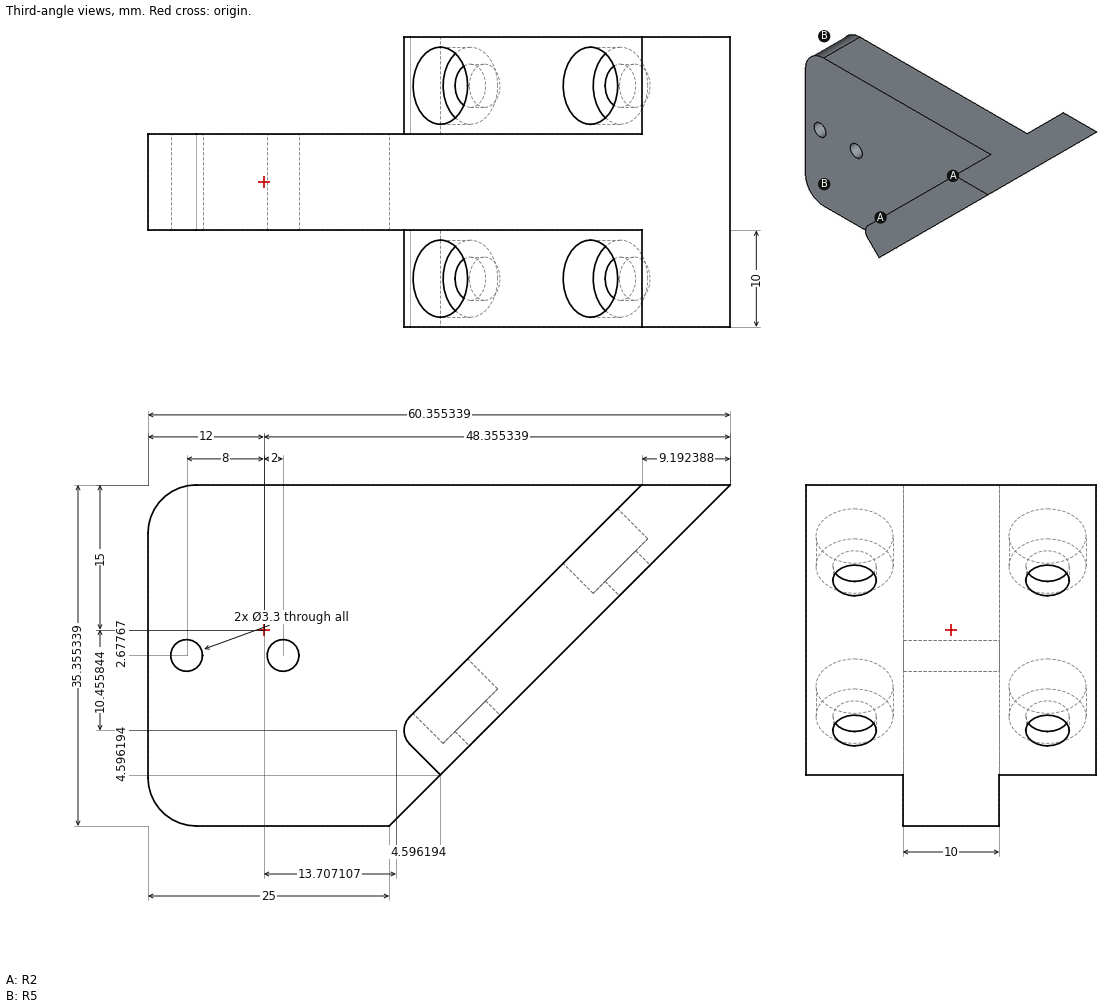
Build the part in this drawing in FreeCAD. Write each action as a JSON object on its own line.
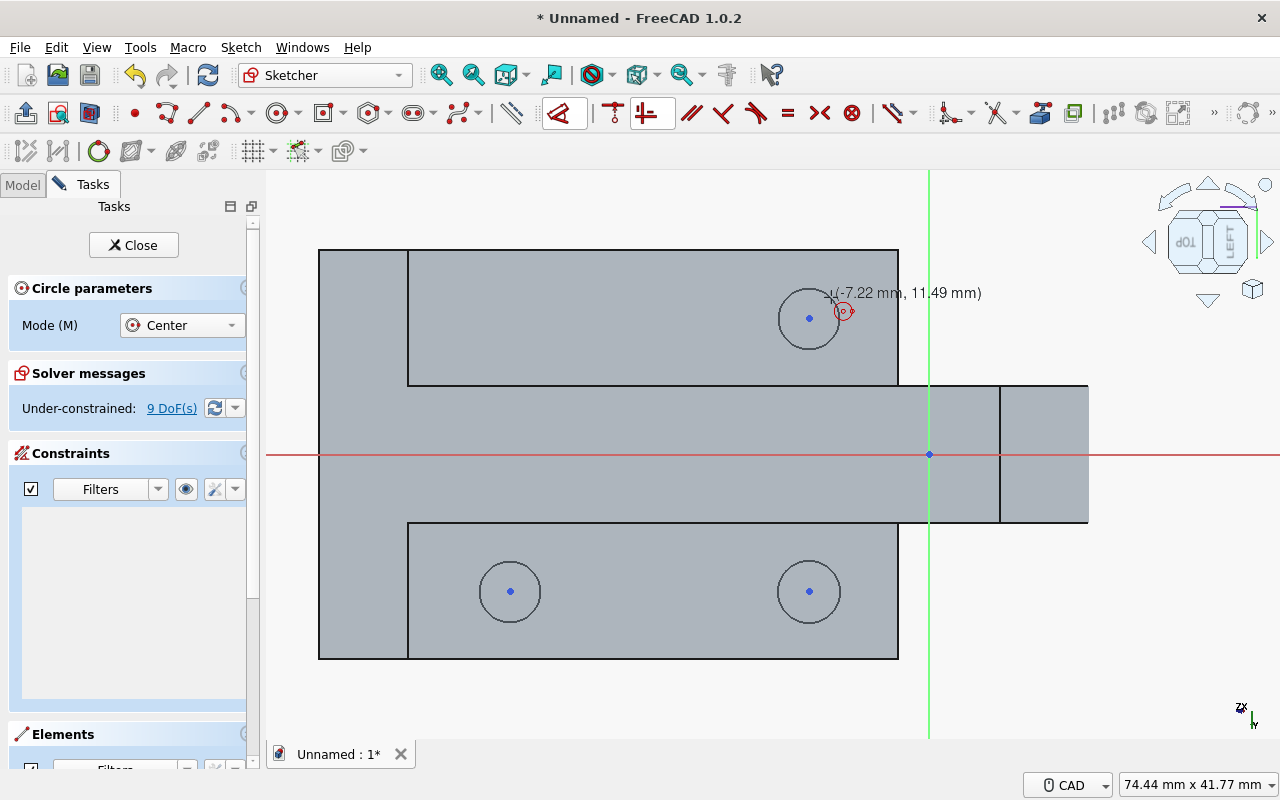
{"action": "left_click", "coordinate": [510, 318]}
{"action": "left_click", "coordinate": [531, 297]}
{"action": "key", "text": "Escape"}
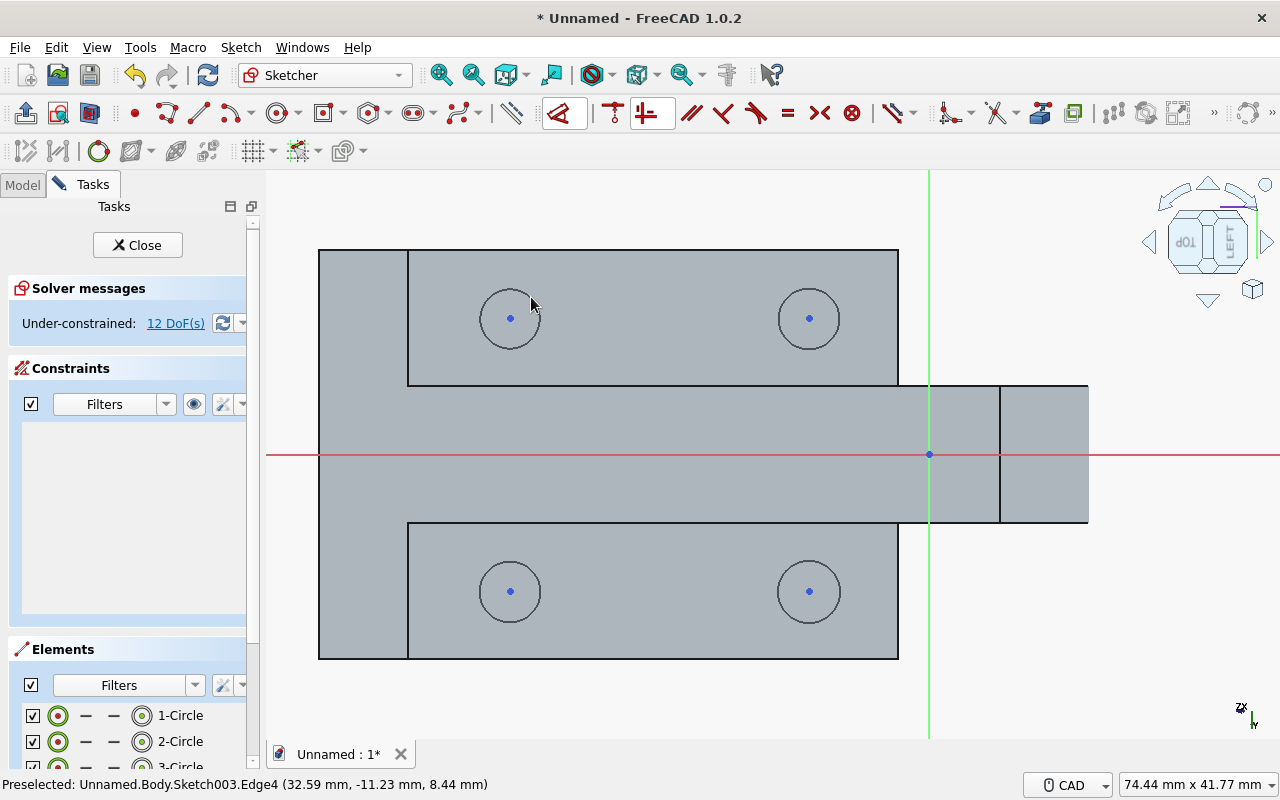
{"action": "left_click", "coordinate": [831, 570]}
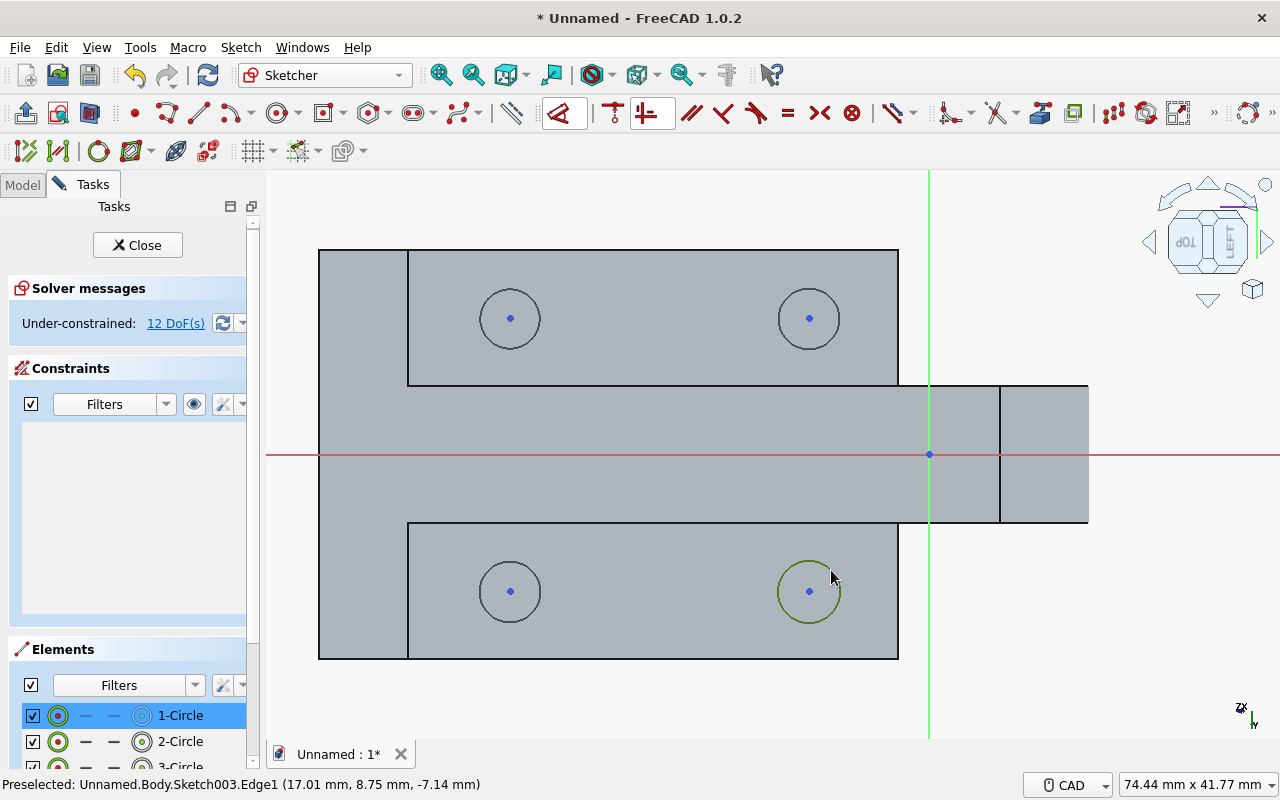
{"action": "left_click", "coordinate": [531, 570]}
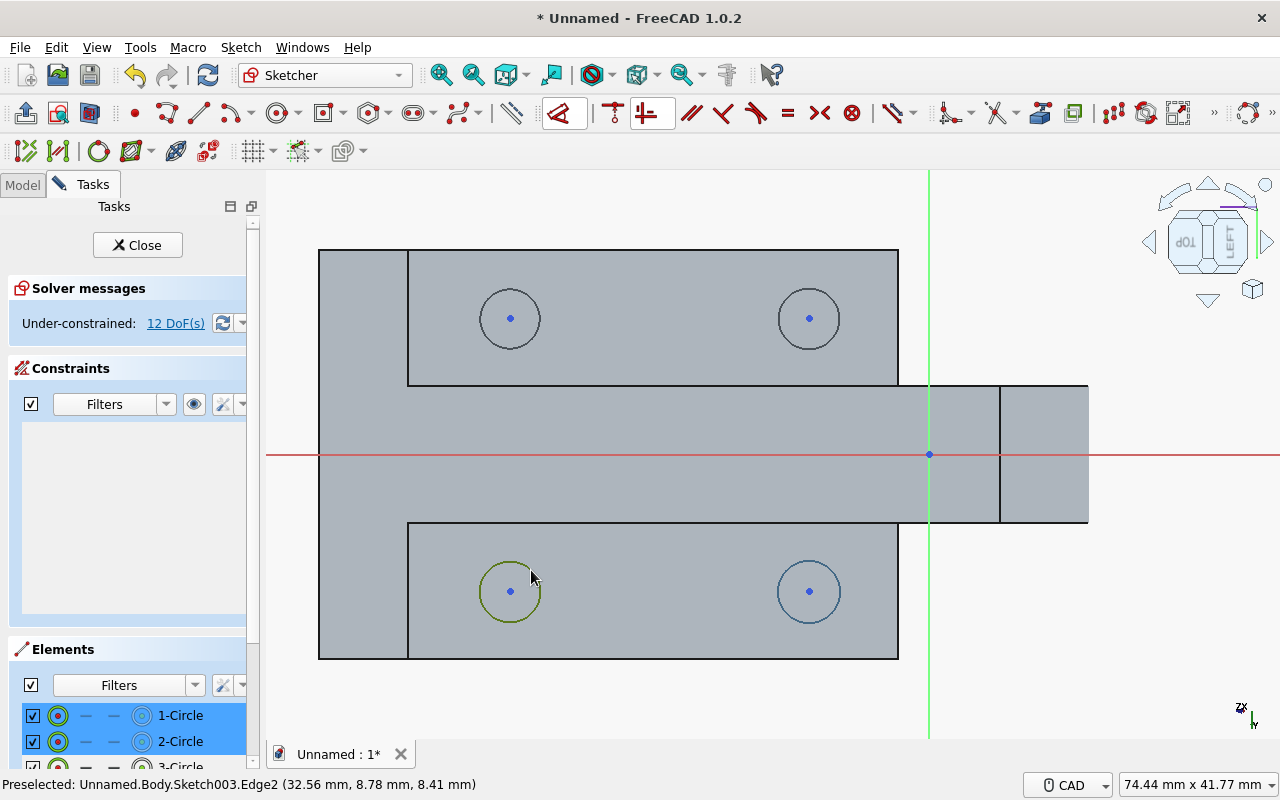
{"action": "left_click", "coordinate": [830, 297]}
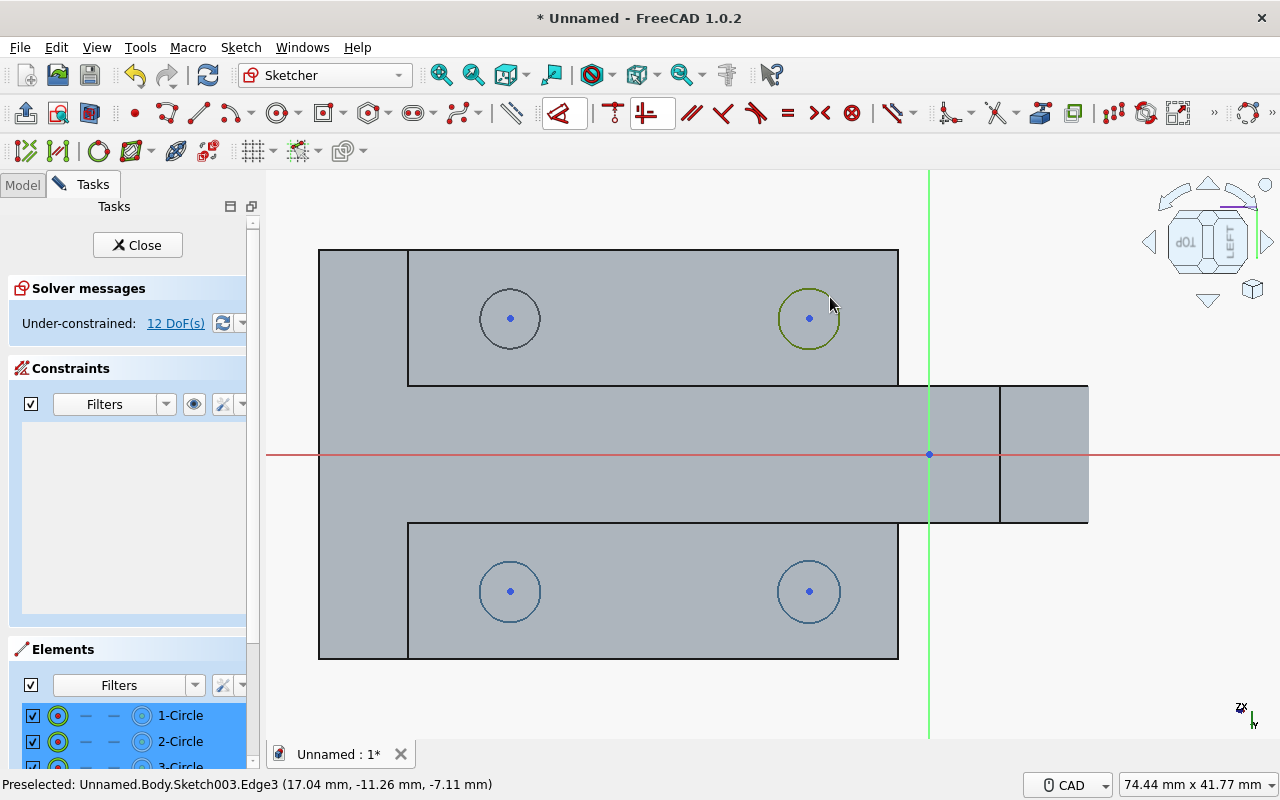
{"action": "left_click", "coordinate": [531, 298]}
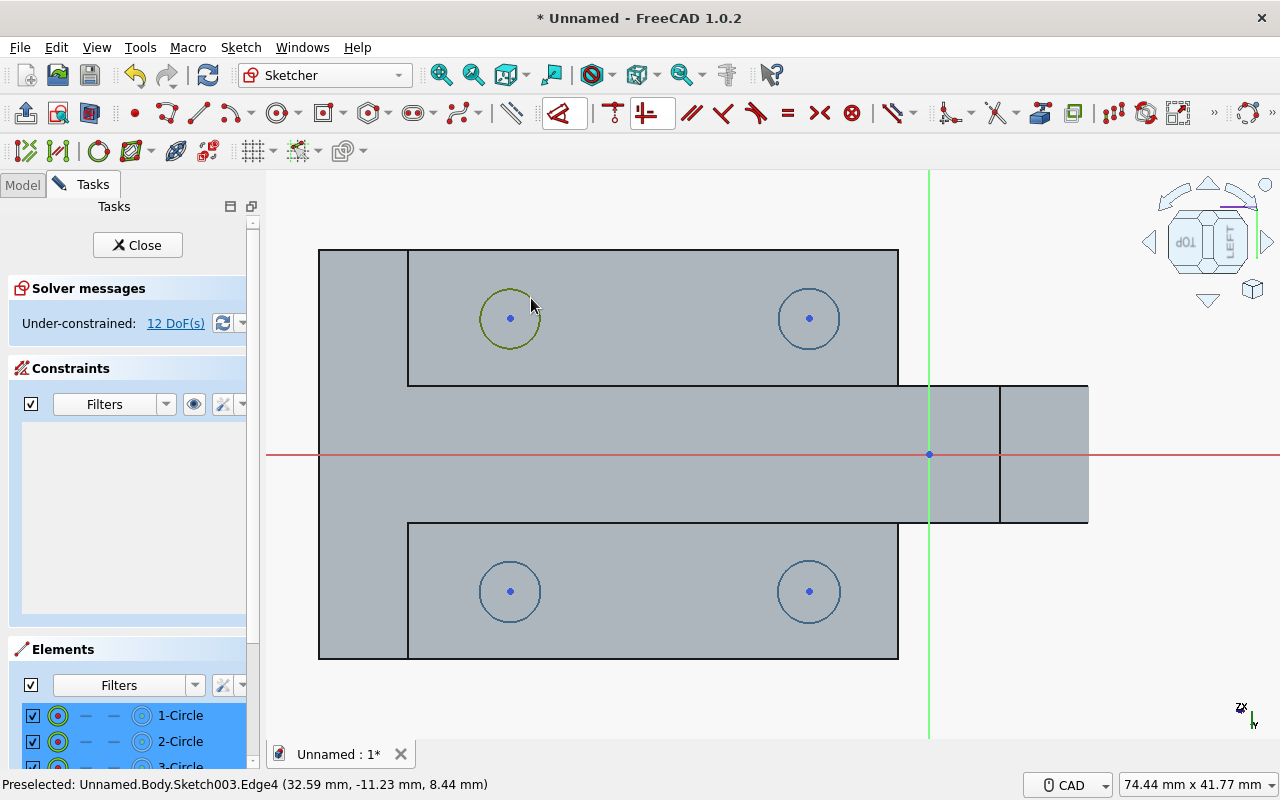
{"action": "left_click", "coordinate": [788, 114]}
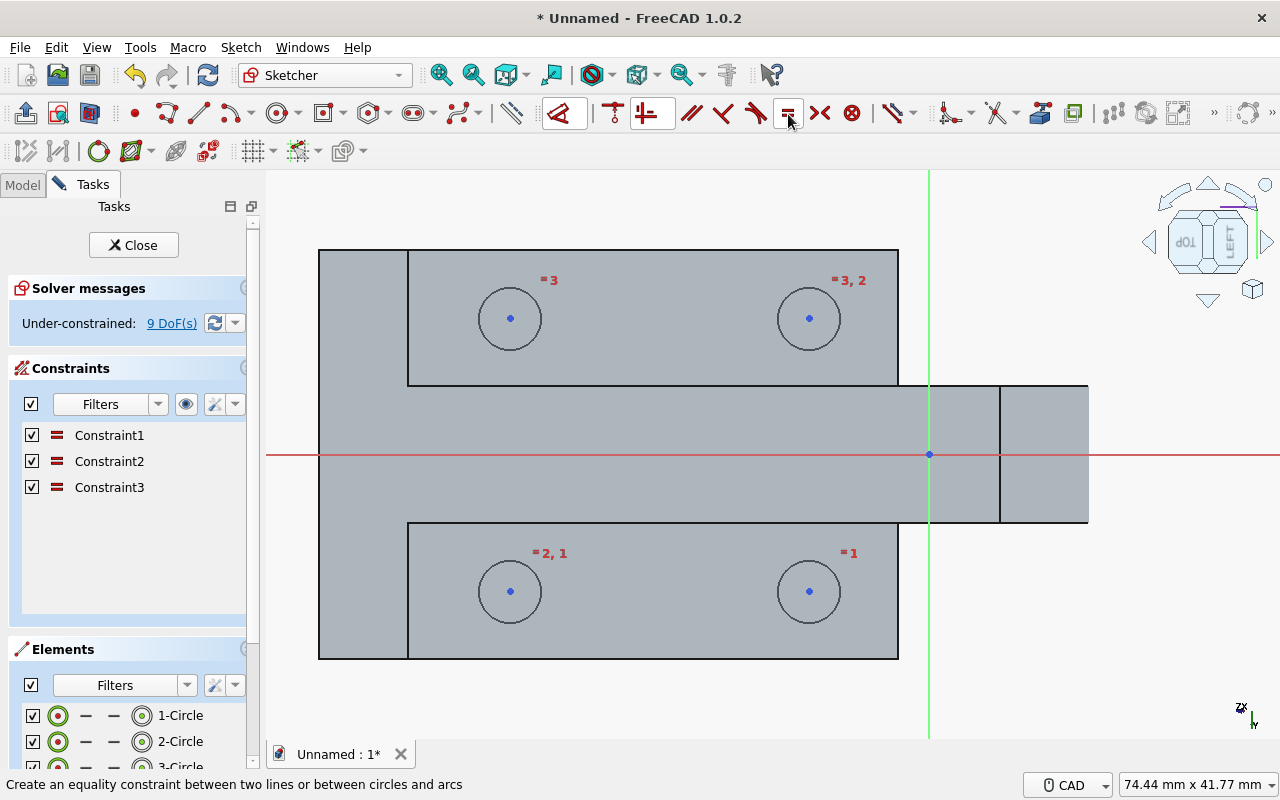
{"action": "left_click", "coordinate": [809, 592]}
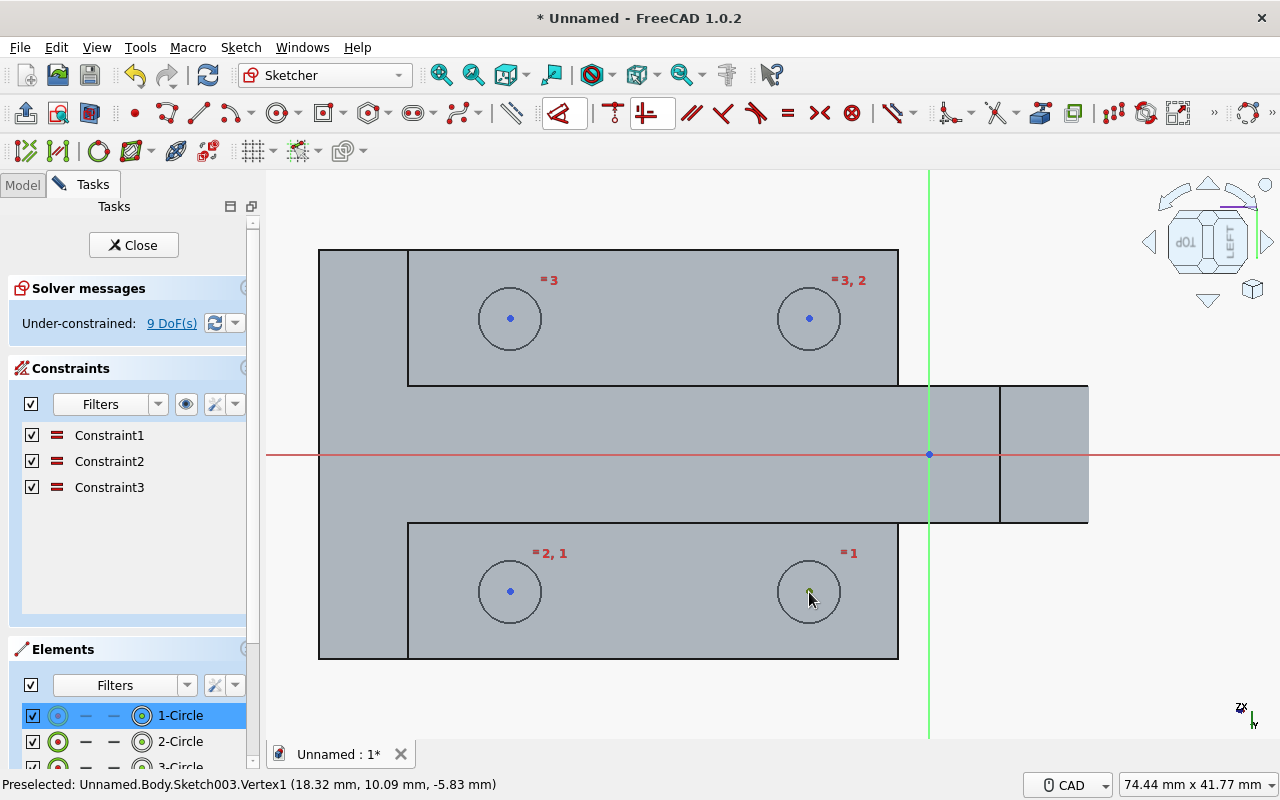
{"action": "left_click", "coordinate": [510, 592]}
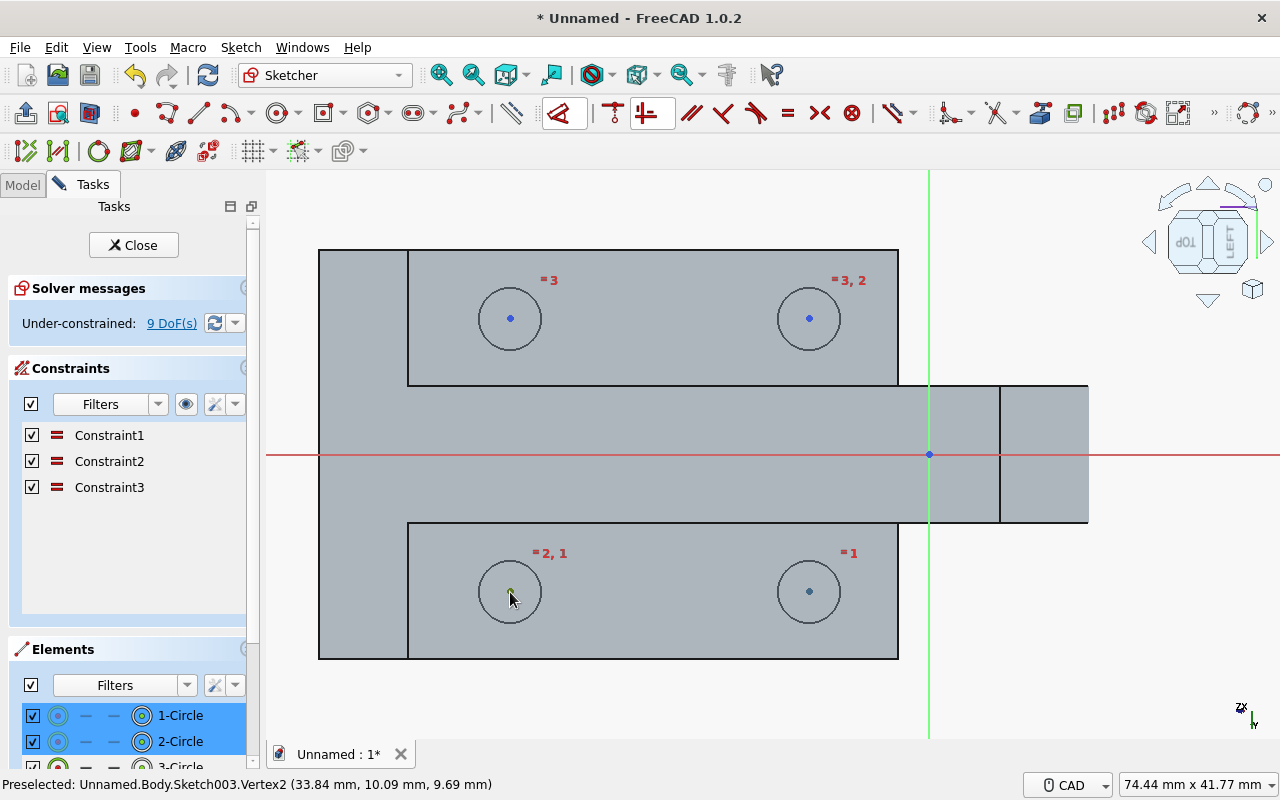
{"action": "key", "text": "h"}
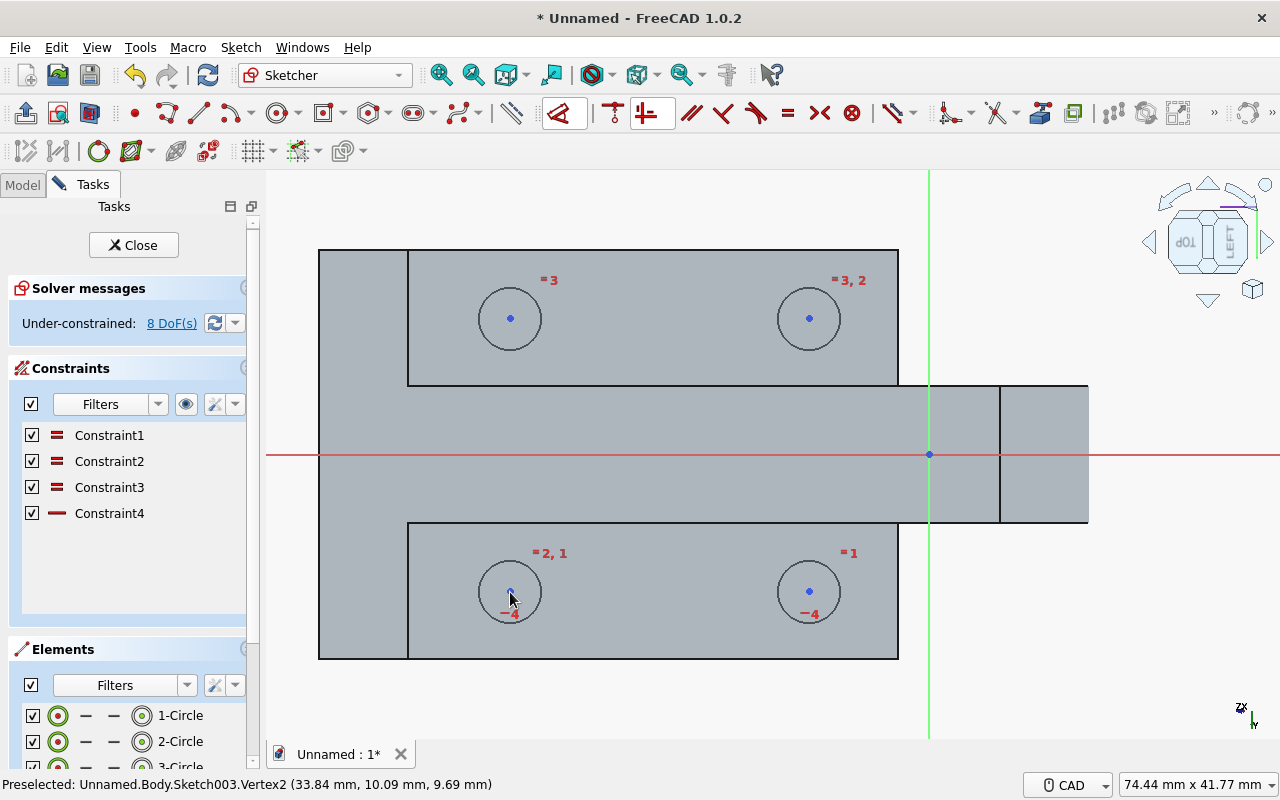
{"action": "left_click", "coordinate": [809, 592]}